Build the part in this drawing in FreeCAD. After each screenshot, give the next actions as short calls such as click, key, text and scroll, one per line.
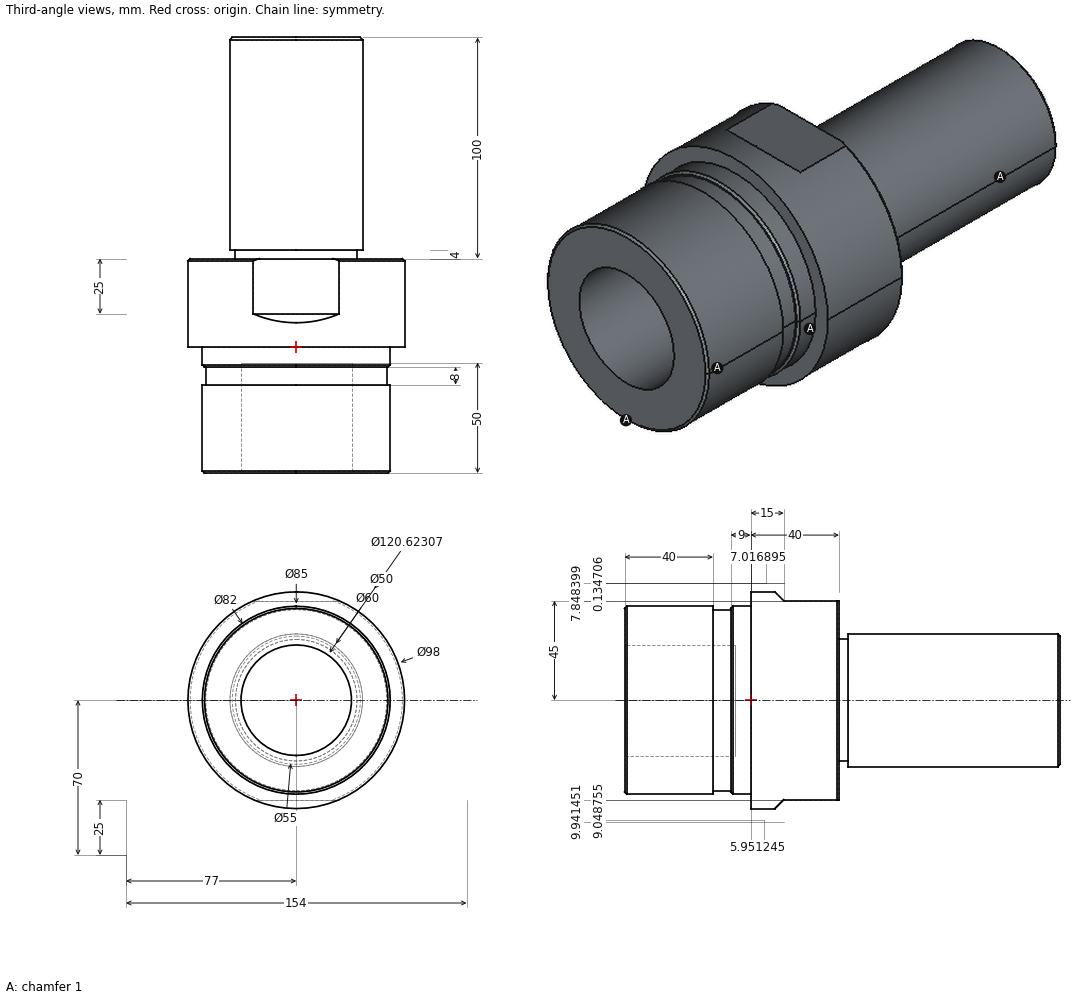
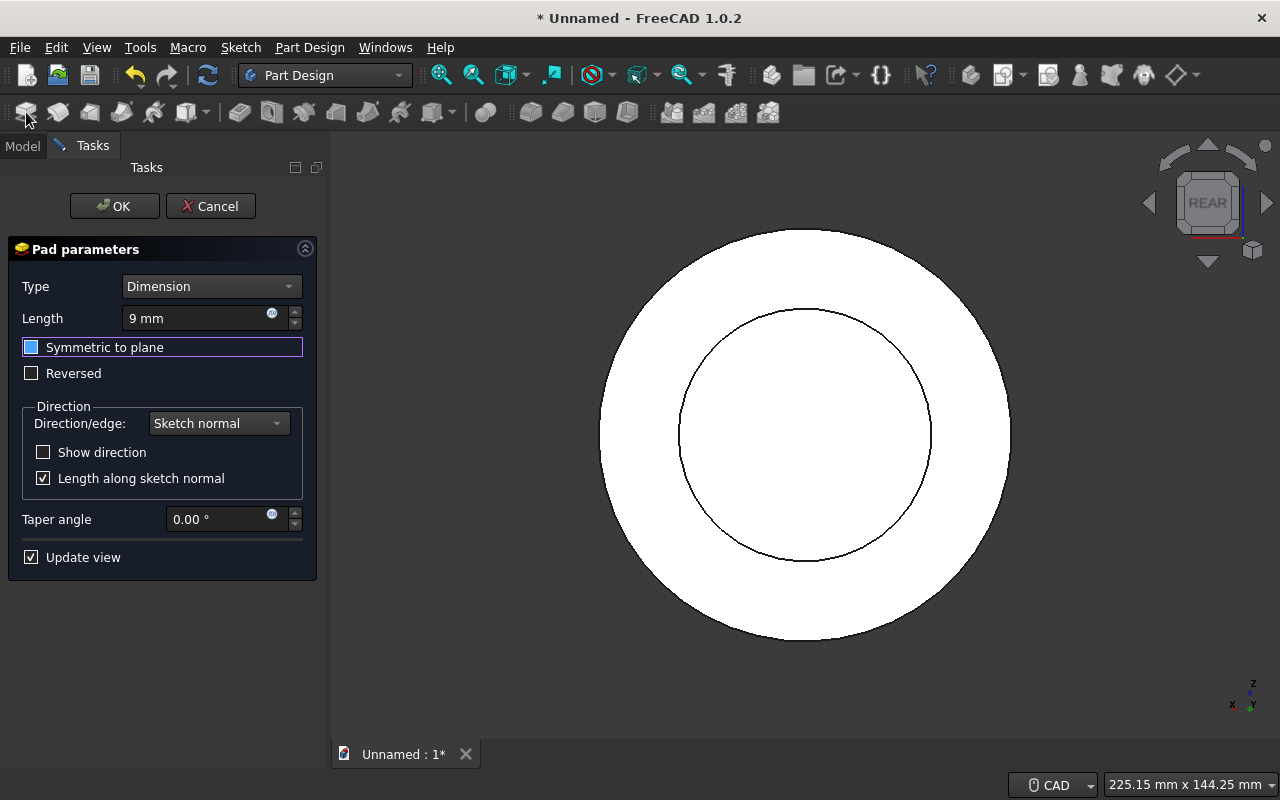
click(115, 206)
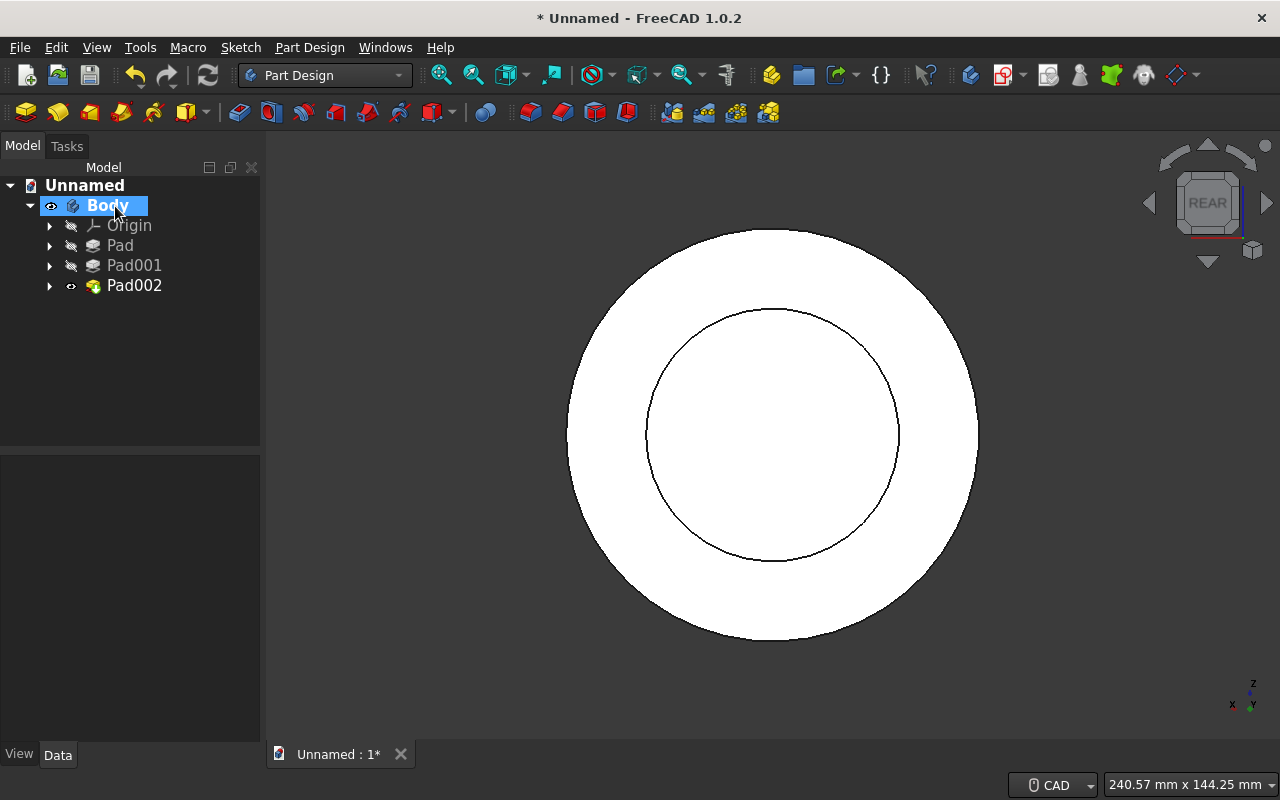
key(0)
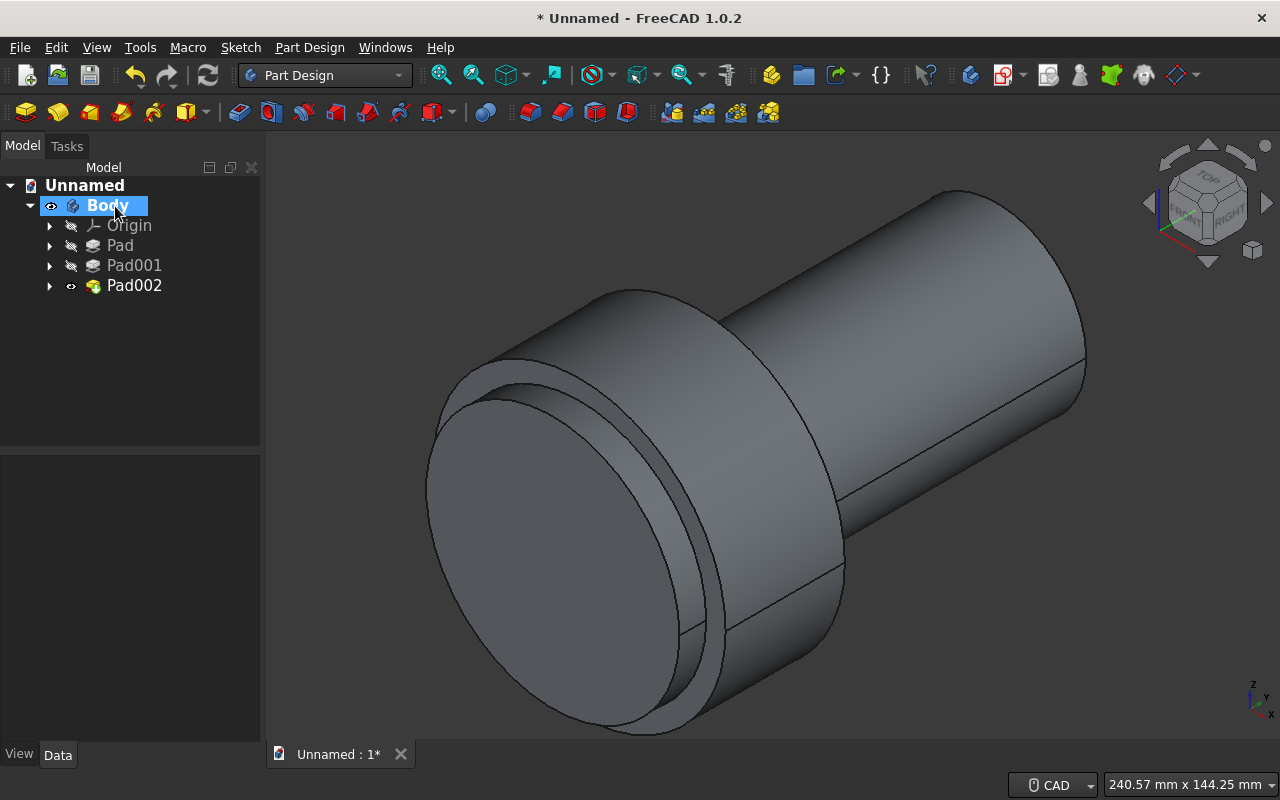
click(442, 76)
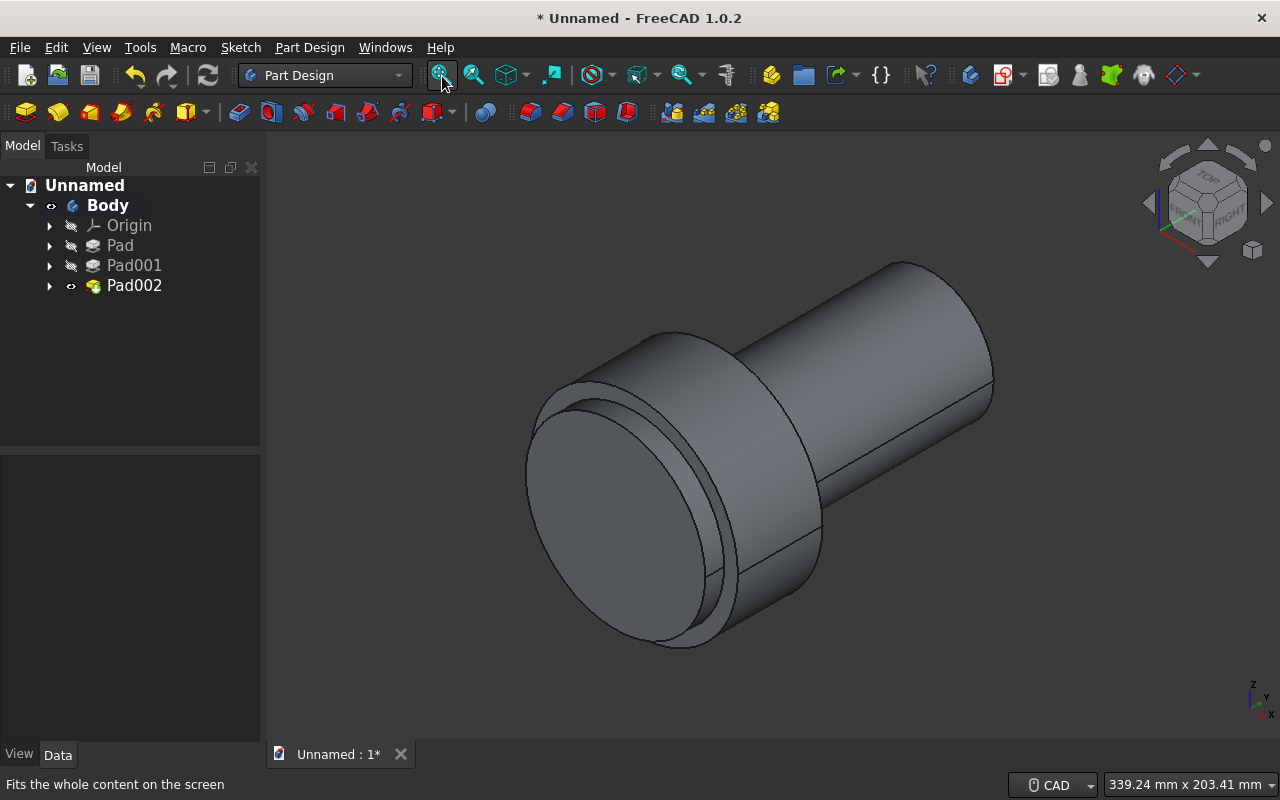
click(615, 525)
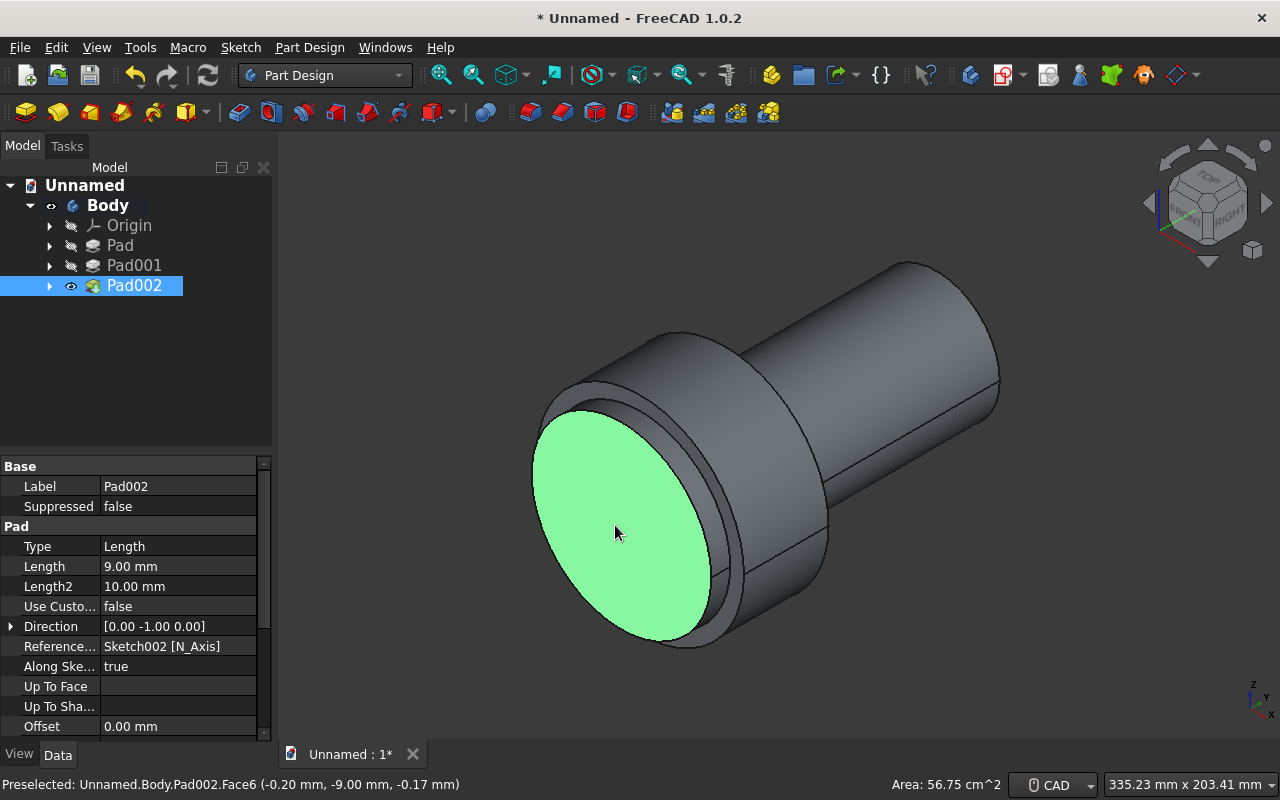
click(1004, 76)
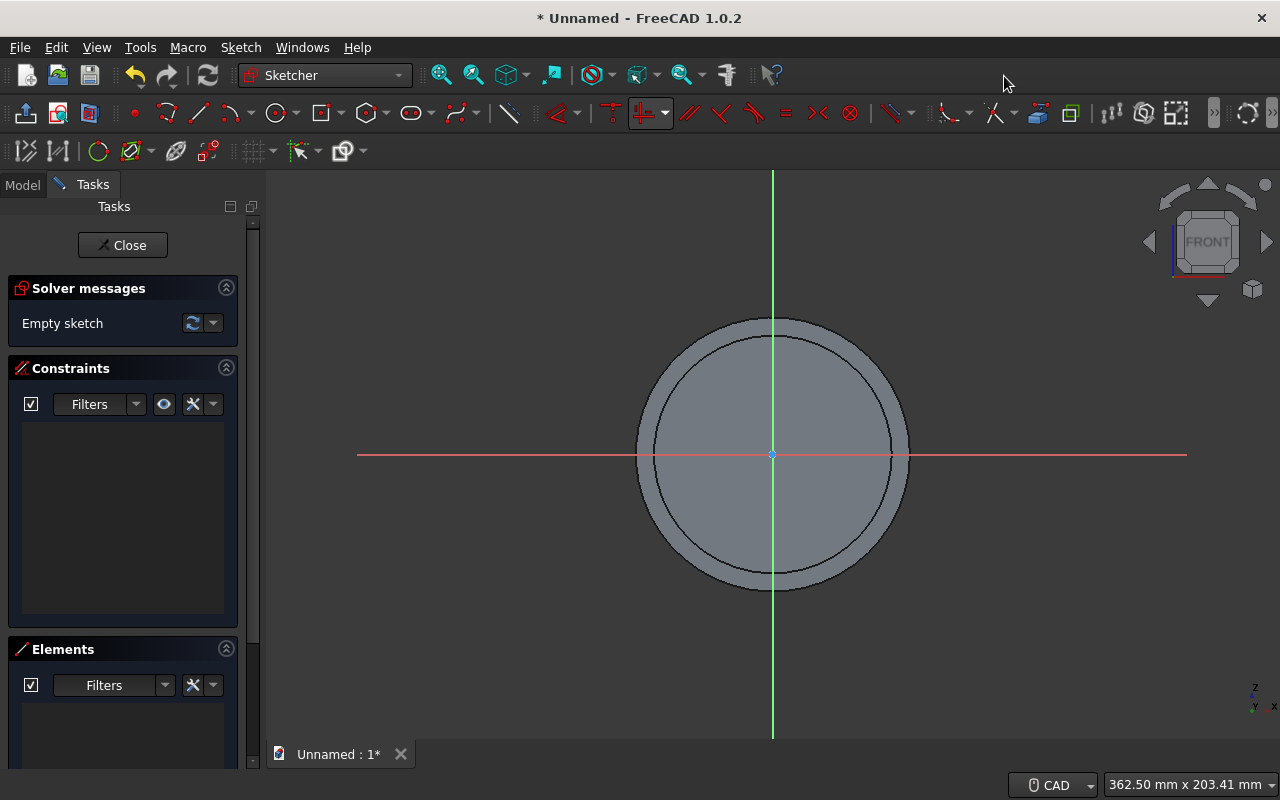
scroll(912, 455, up, 2)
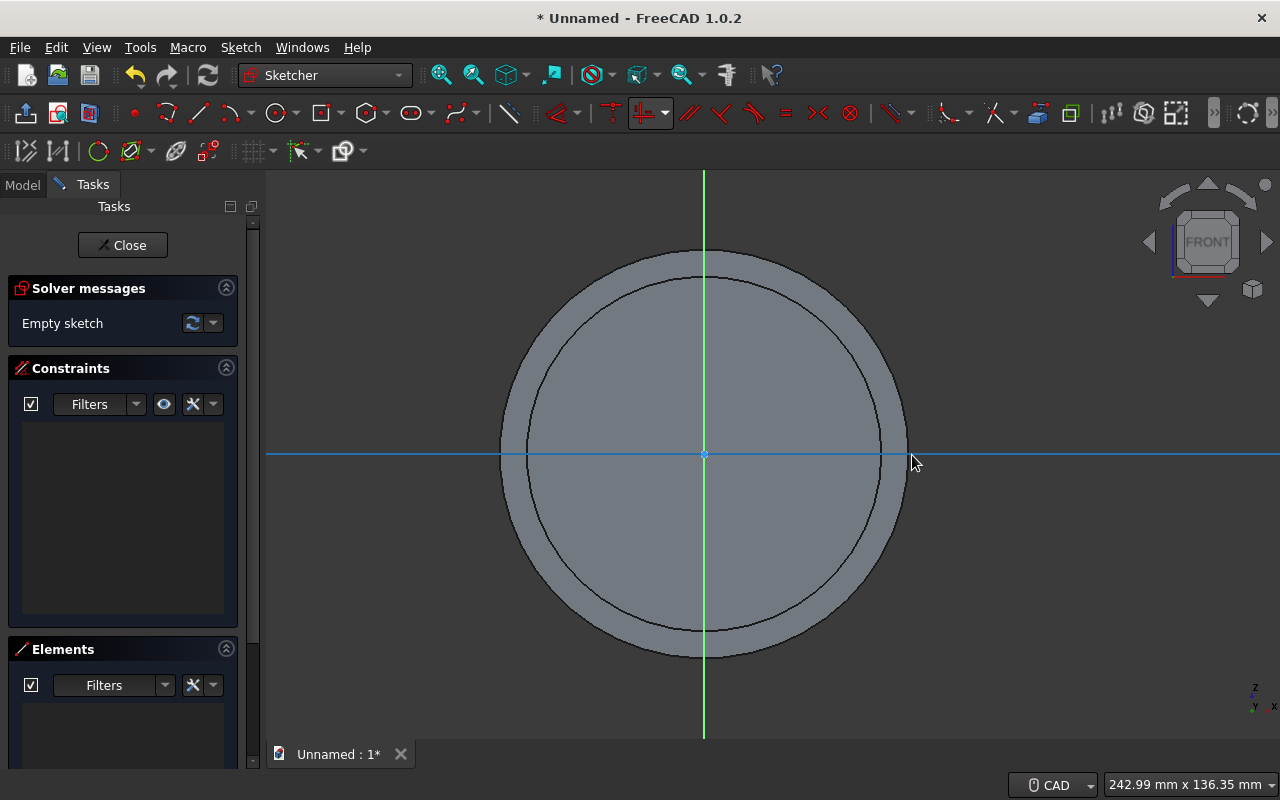
click(276, 114)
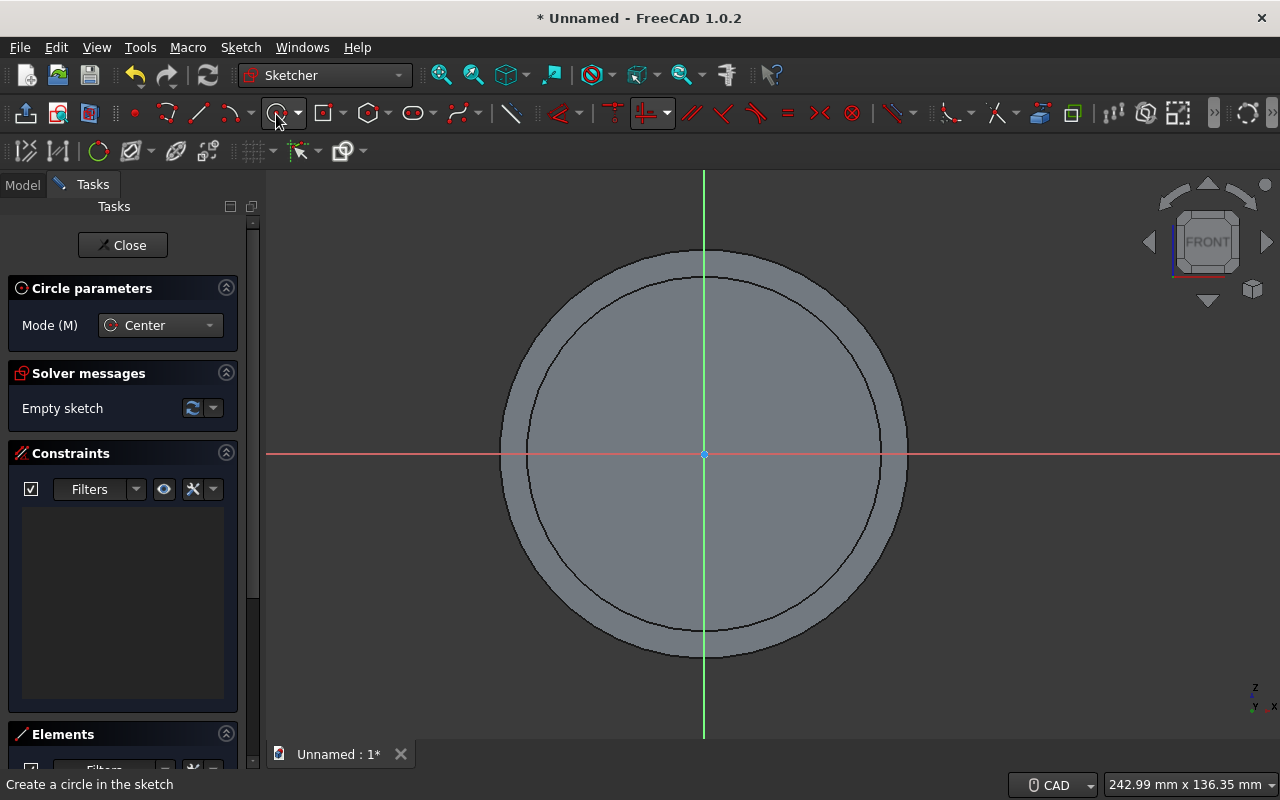
click(704, 454)
click(825, 333)
key(Escape)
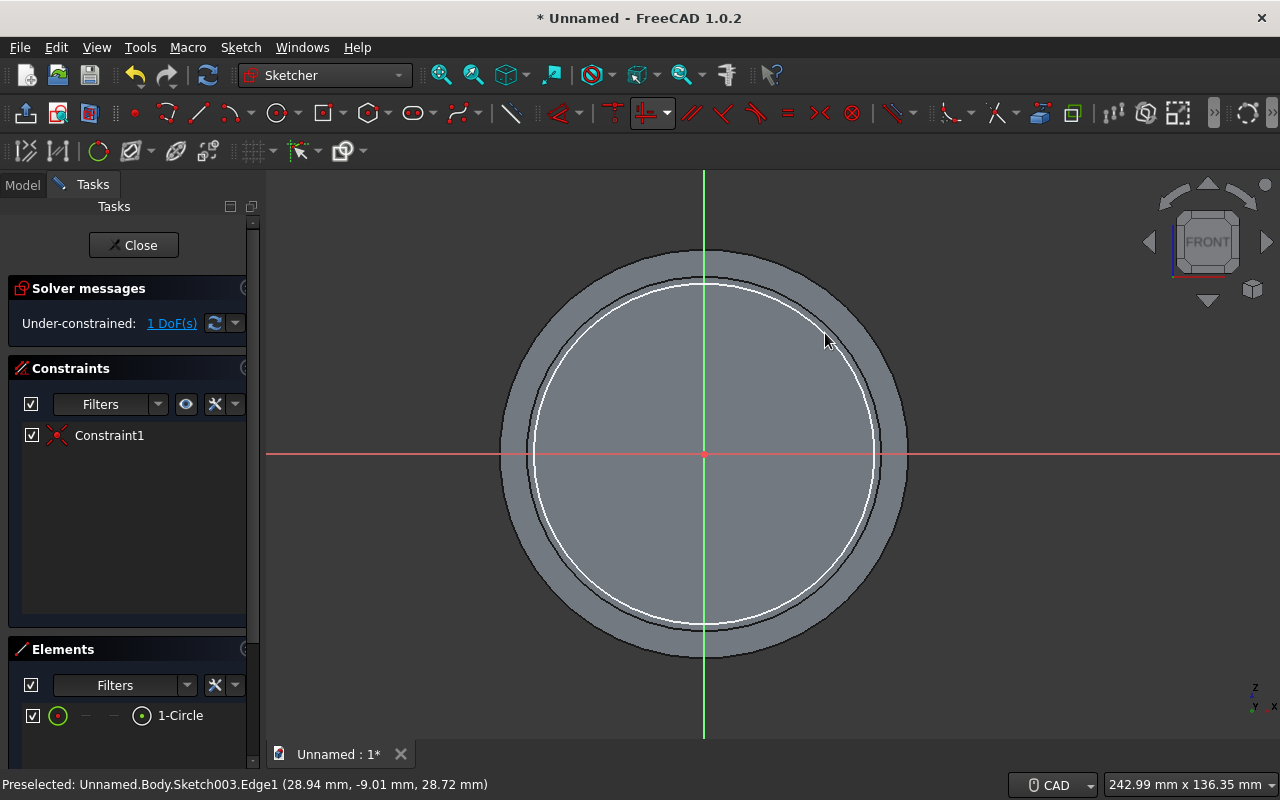
click(558, 114)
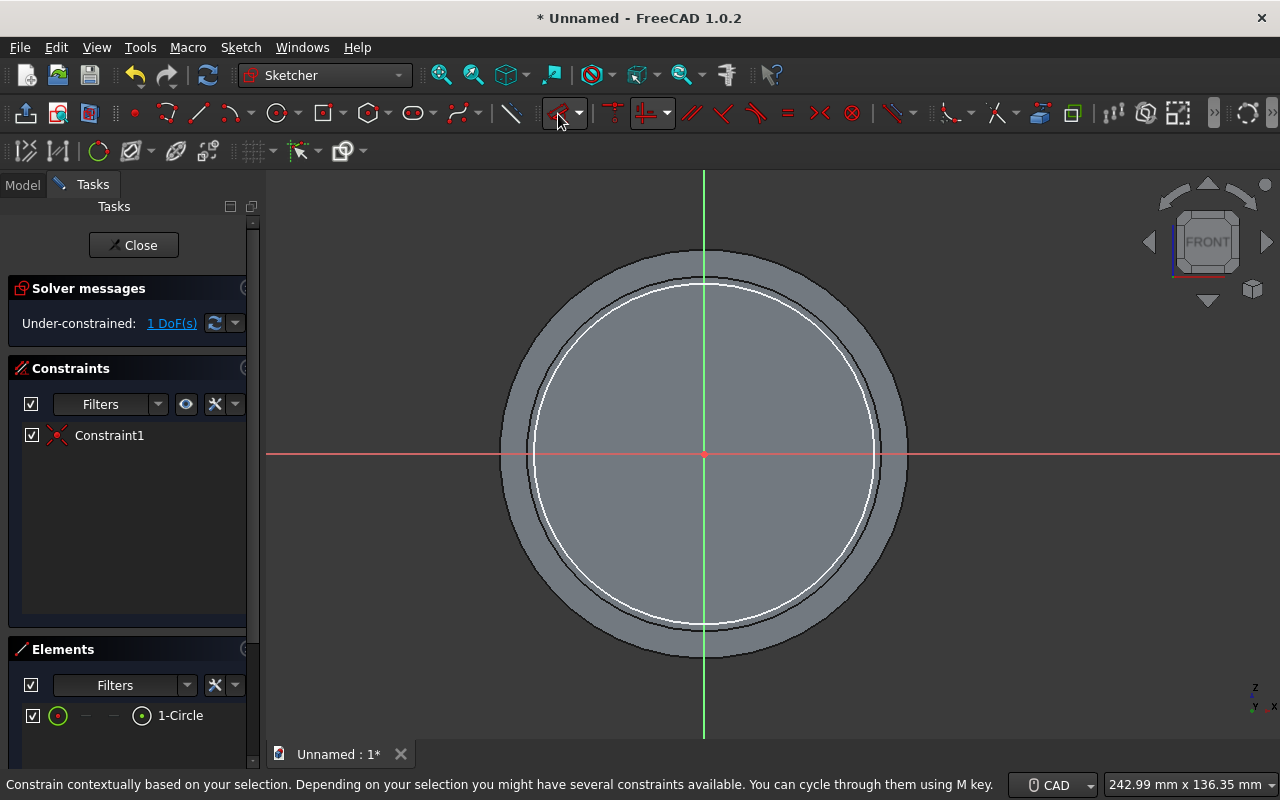
click(824, 333)
click(847, 310)